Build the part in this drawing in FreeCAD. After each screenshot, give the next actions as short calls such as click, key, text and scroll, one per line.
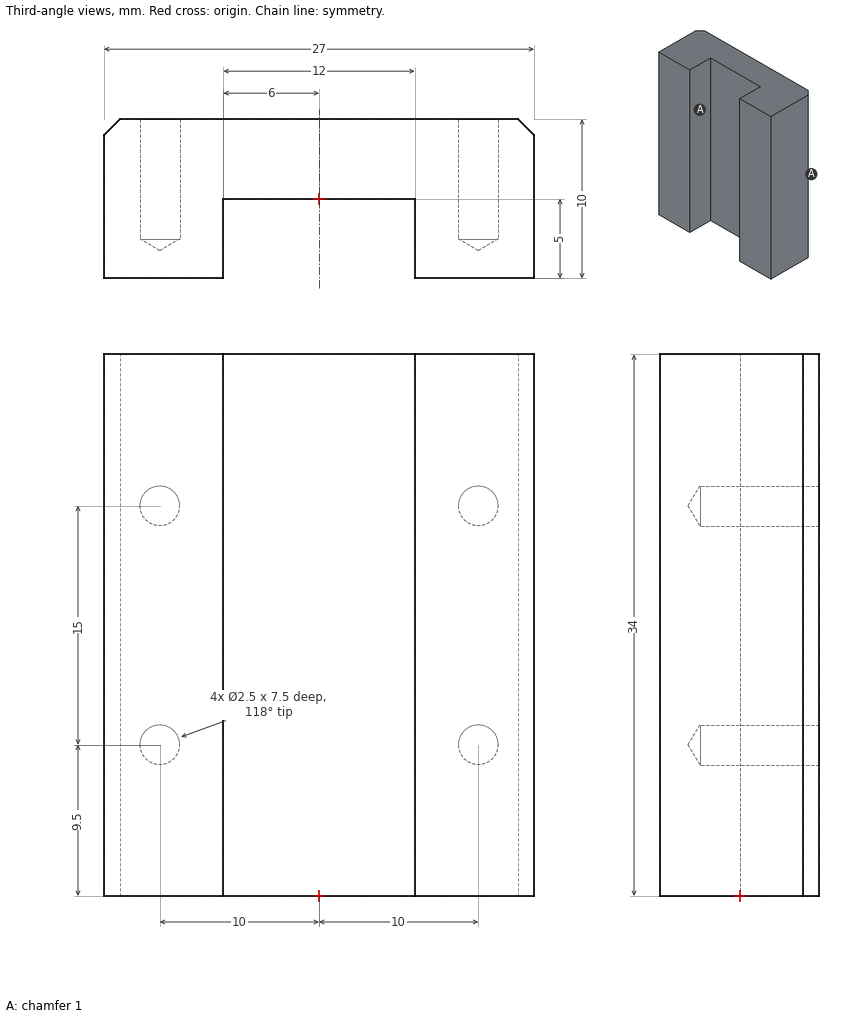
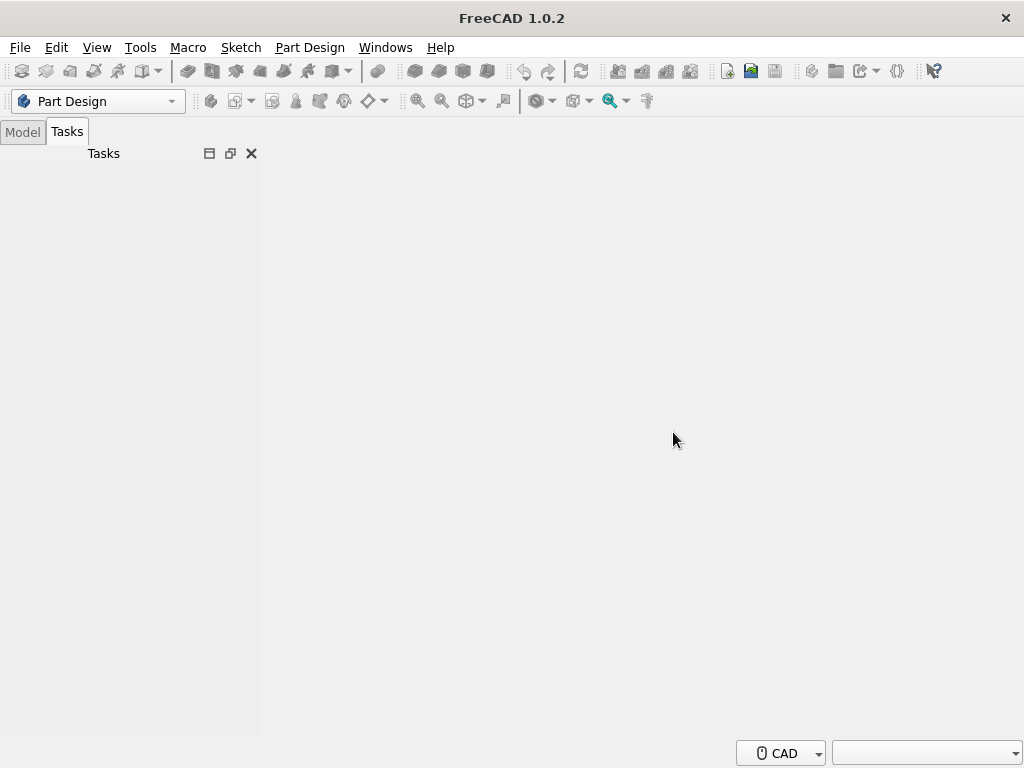
key(ctrl+n)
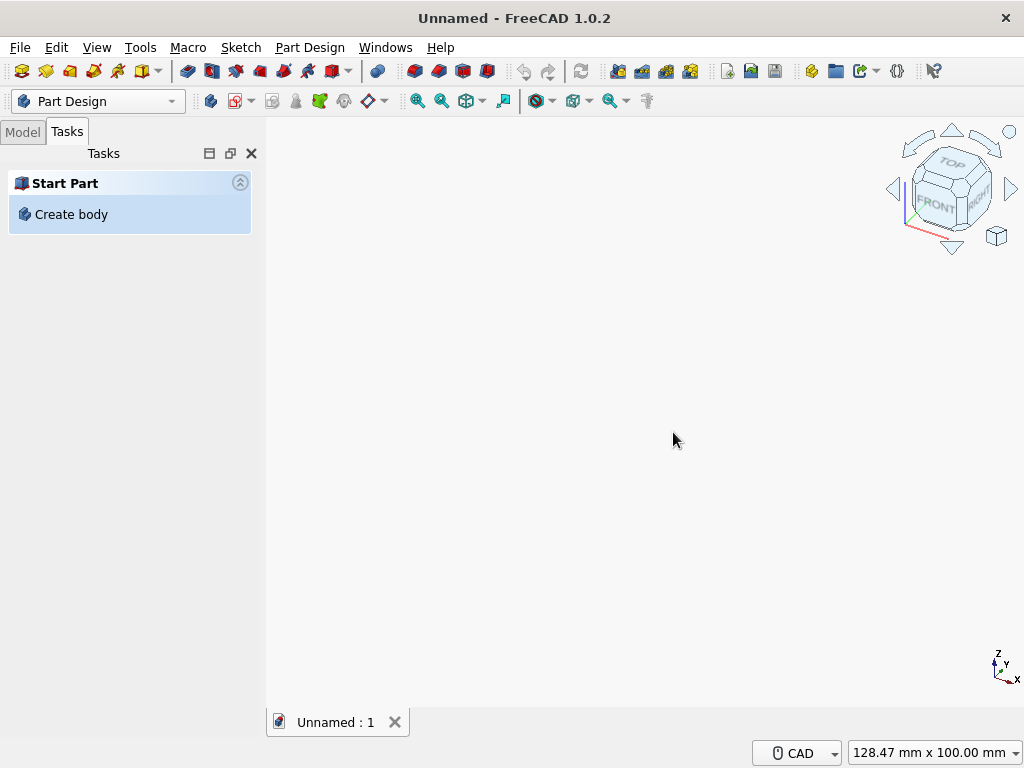
click(236, 102)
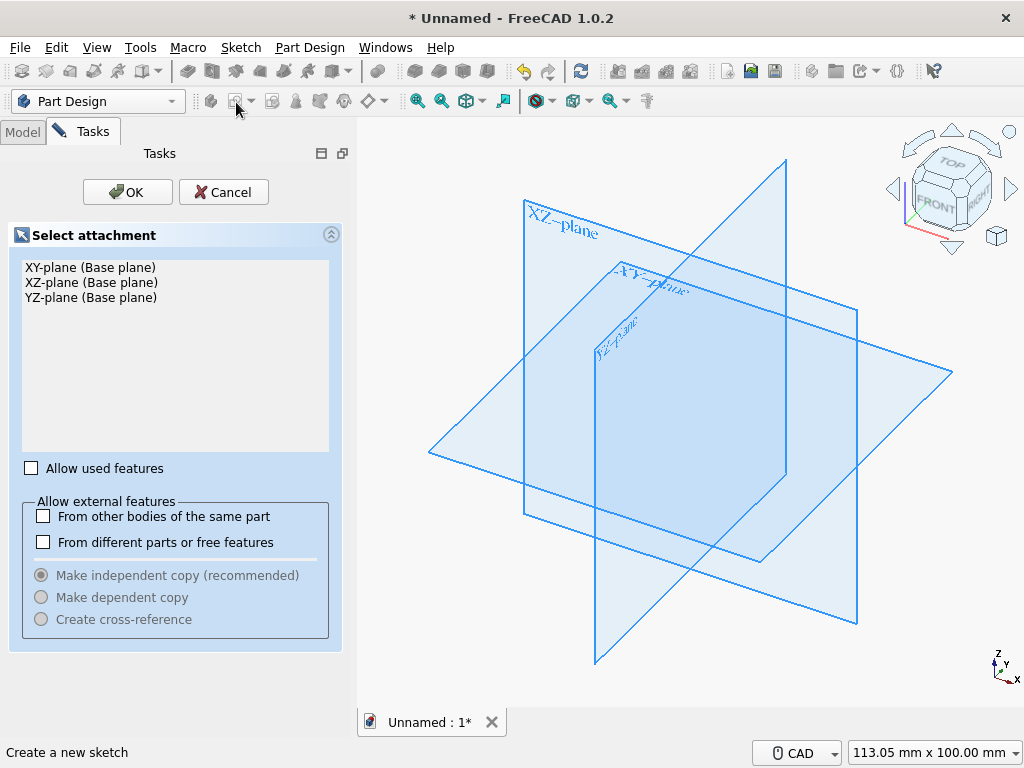
click(82, 268)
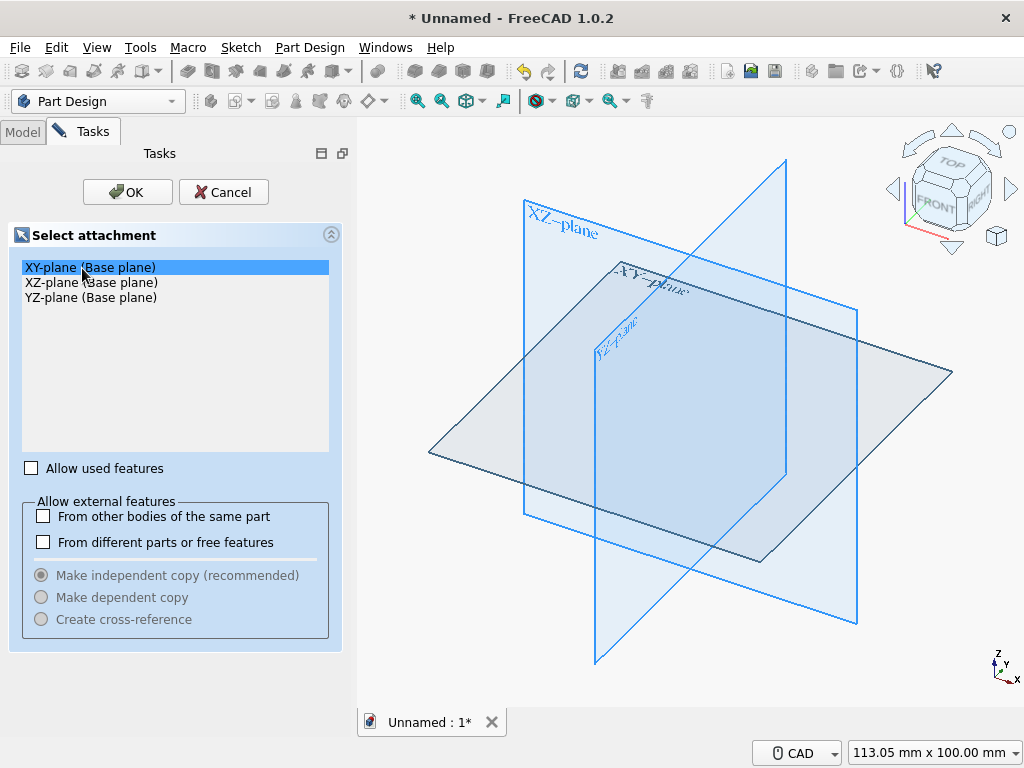
click(128, 192)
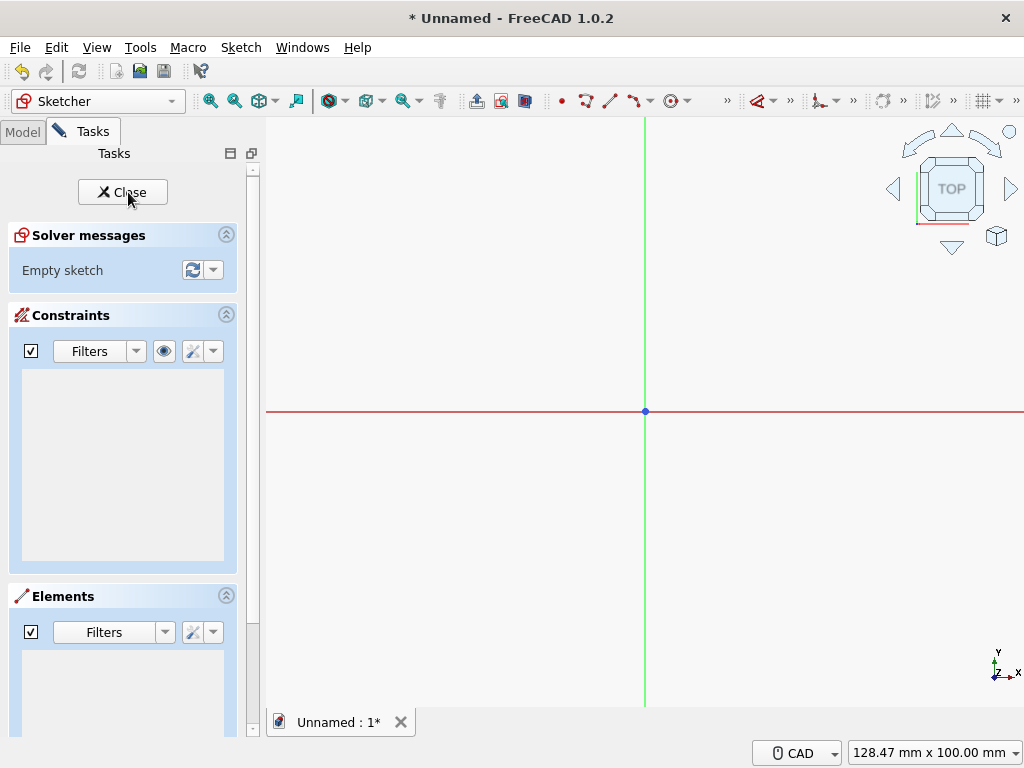
scroll(685, 412, up, 5)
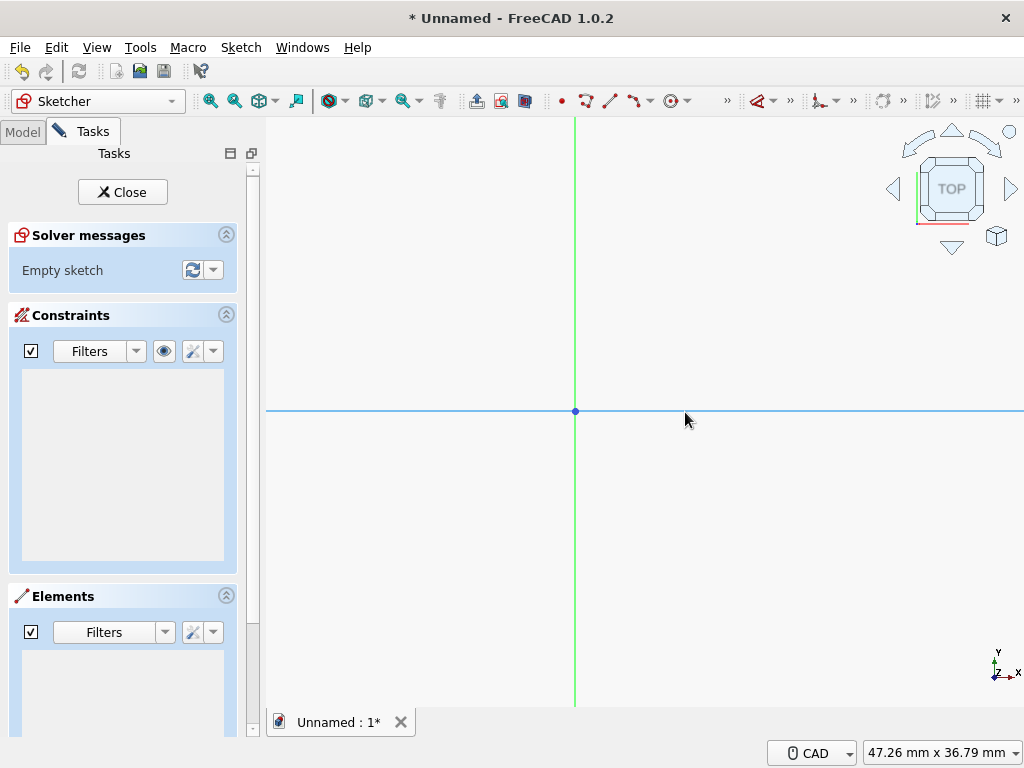
click(586, 102)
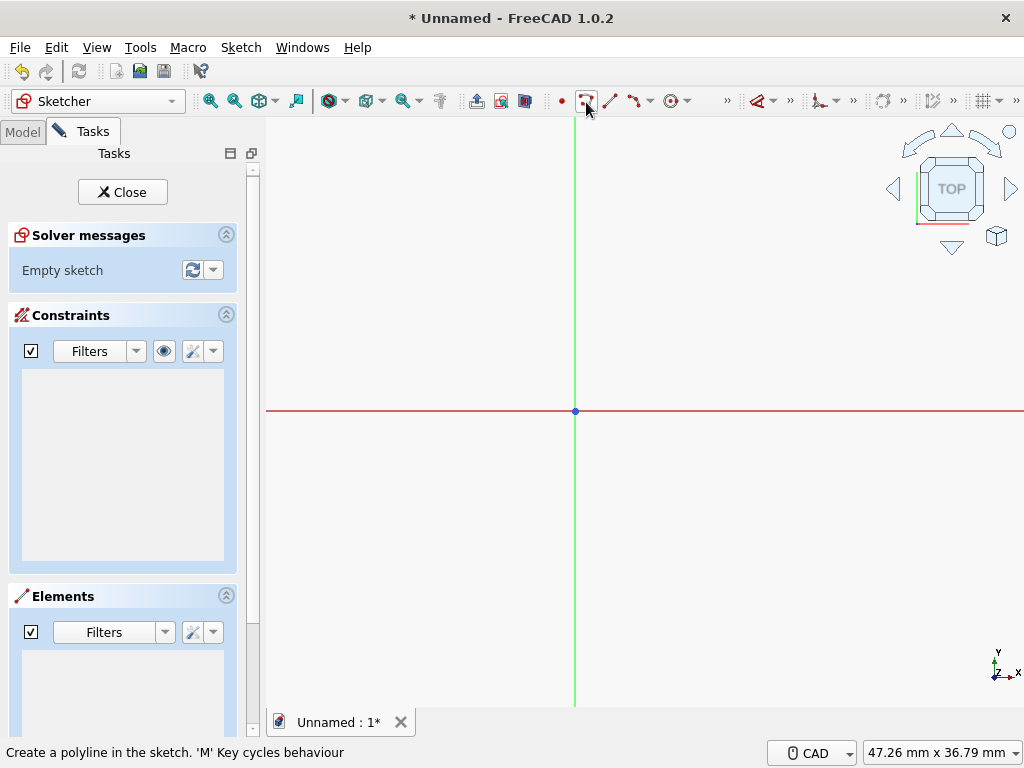
click(479, 411)
click(672, 402)
click(672, 491)
click(792, 491)
click(792, 331)
click(359, 331)
click(359, 491)
click(479, 491)
click(479, 411)
key(Escape)
key(Escape)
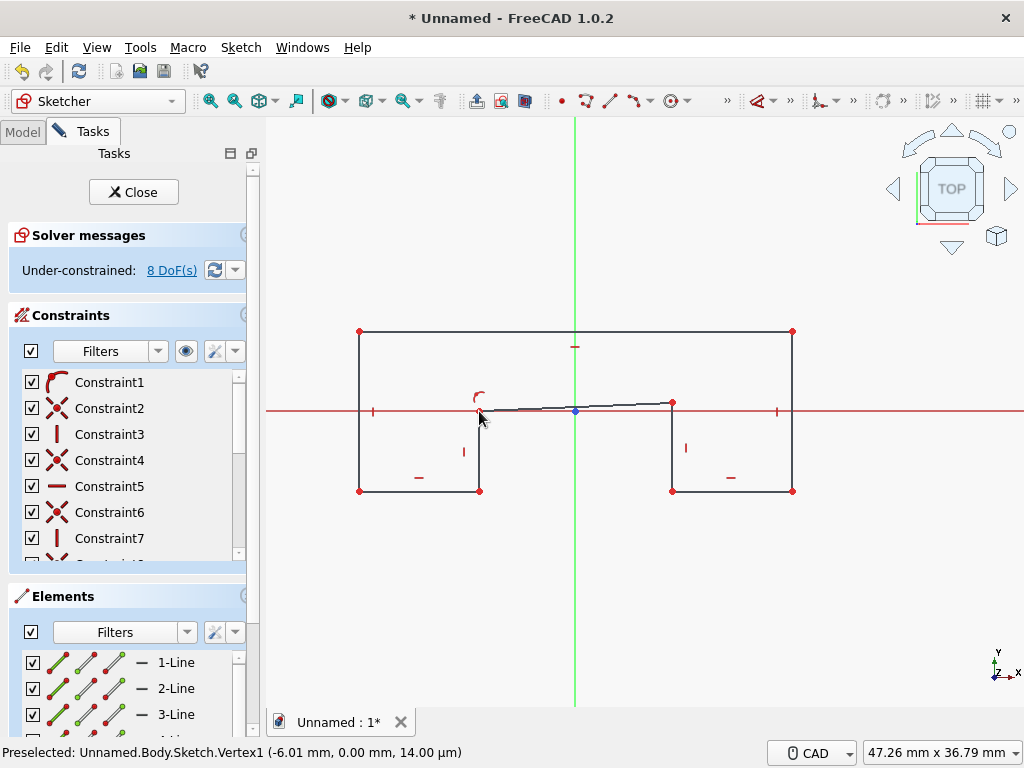
click(537, 409)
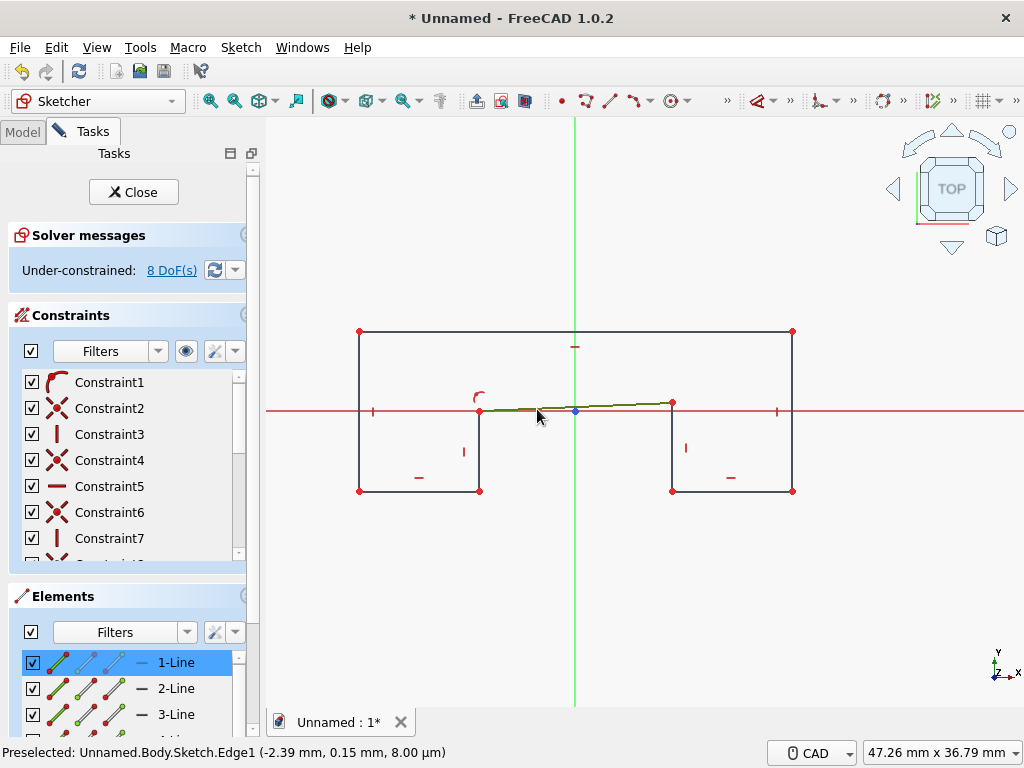
key(h)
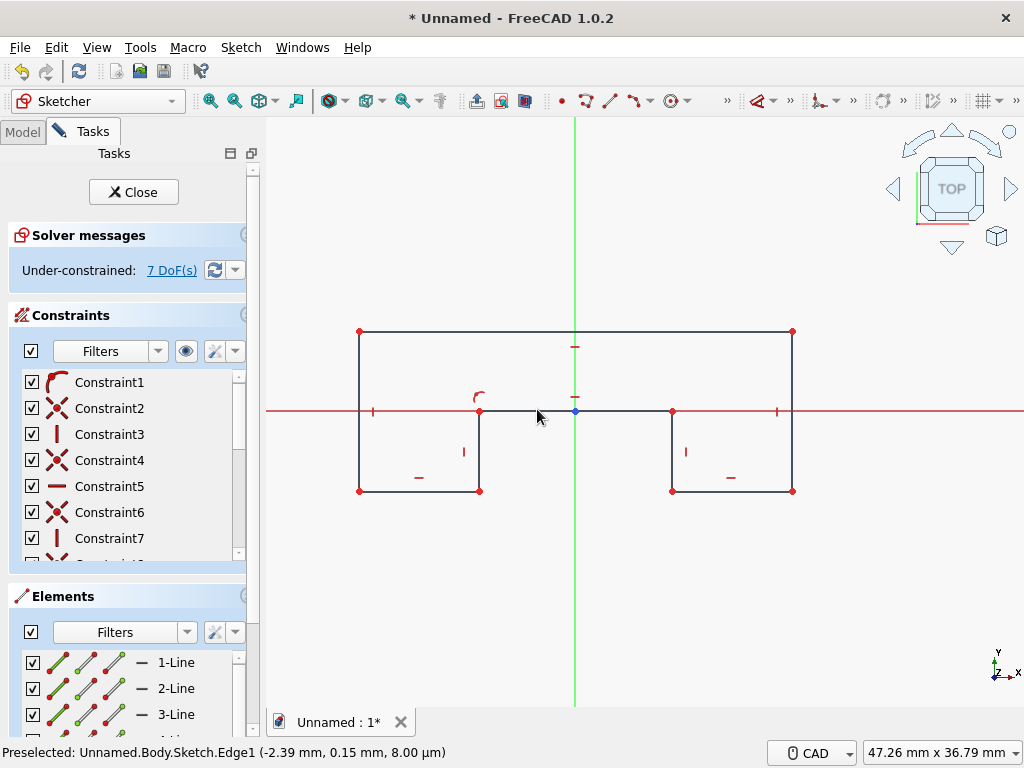
click(792, 492)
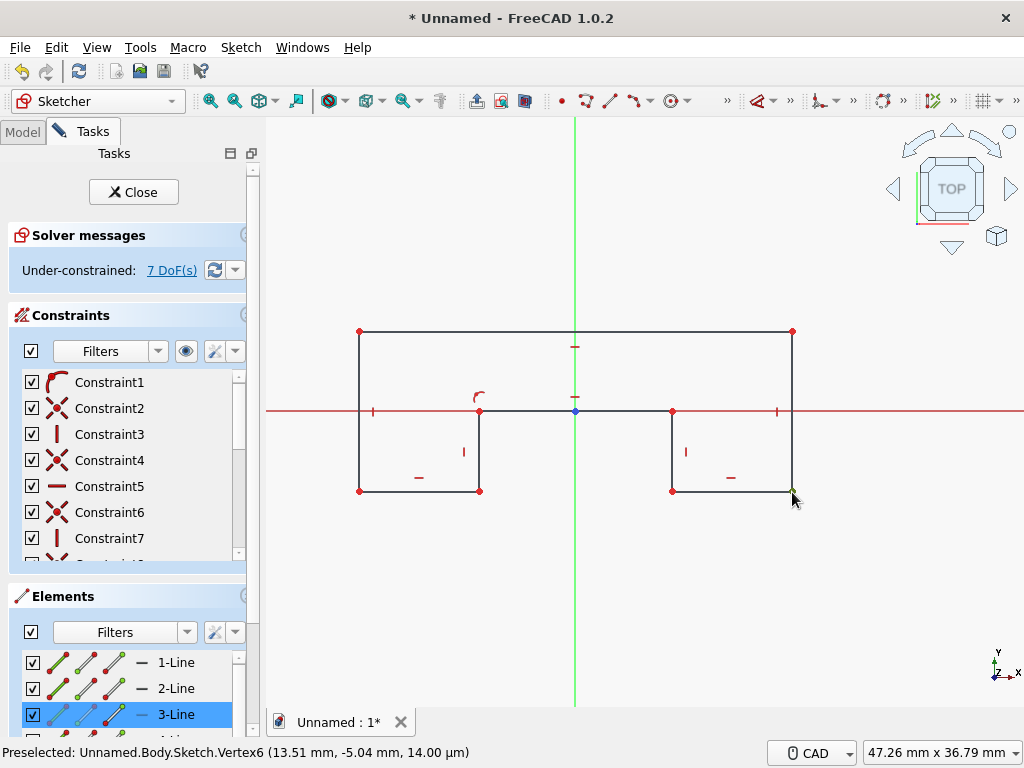
click(359, 492)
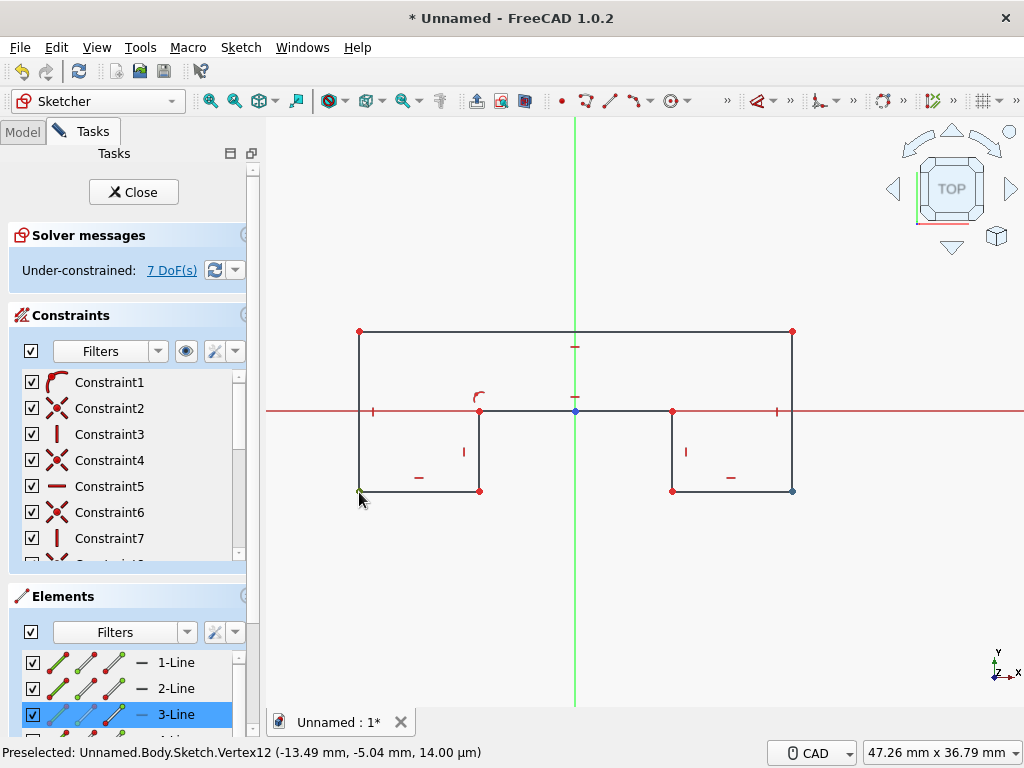
click(575, 641)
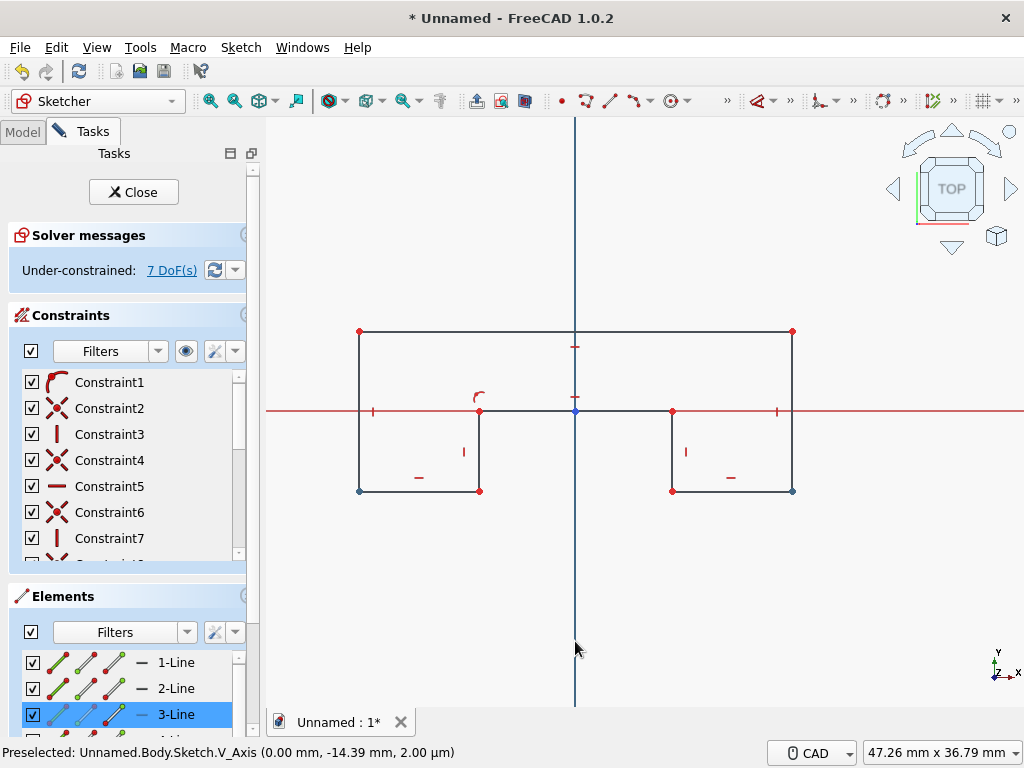
key(s)